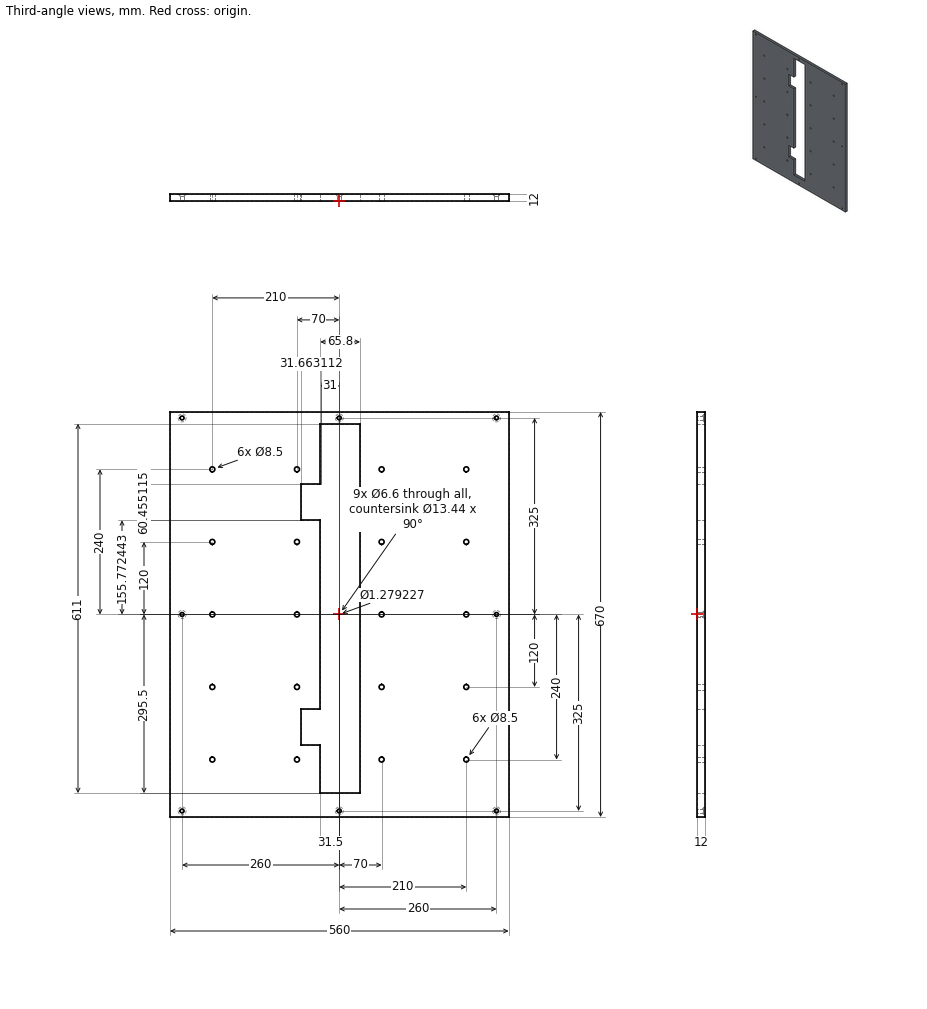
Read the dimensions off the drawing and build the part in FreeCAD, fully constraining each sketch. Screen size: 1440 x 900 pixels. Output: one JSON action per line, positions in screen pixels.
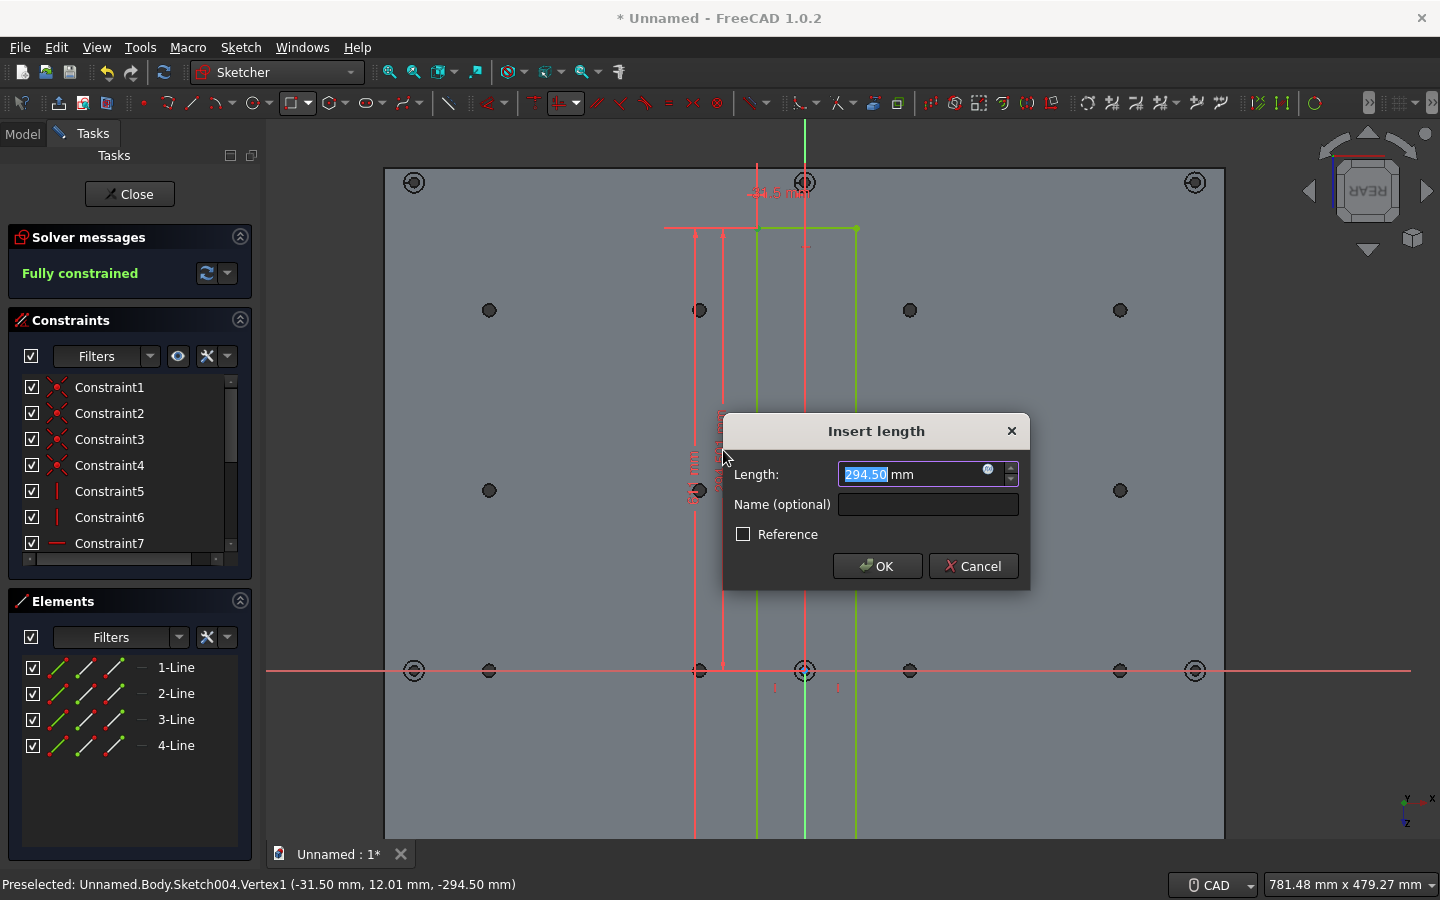
{"action": "type", "text": "295.5"}
{"action": "key", "text": "Return"}
{"action": "key", "text": "Escape"}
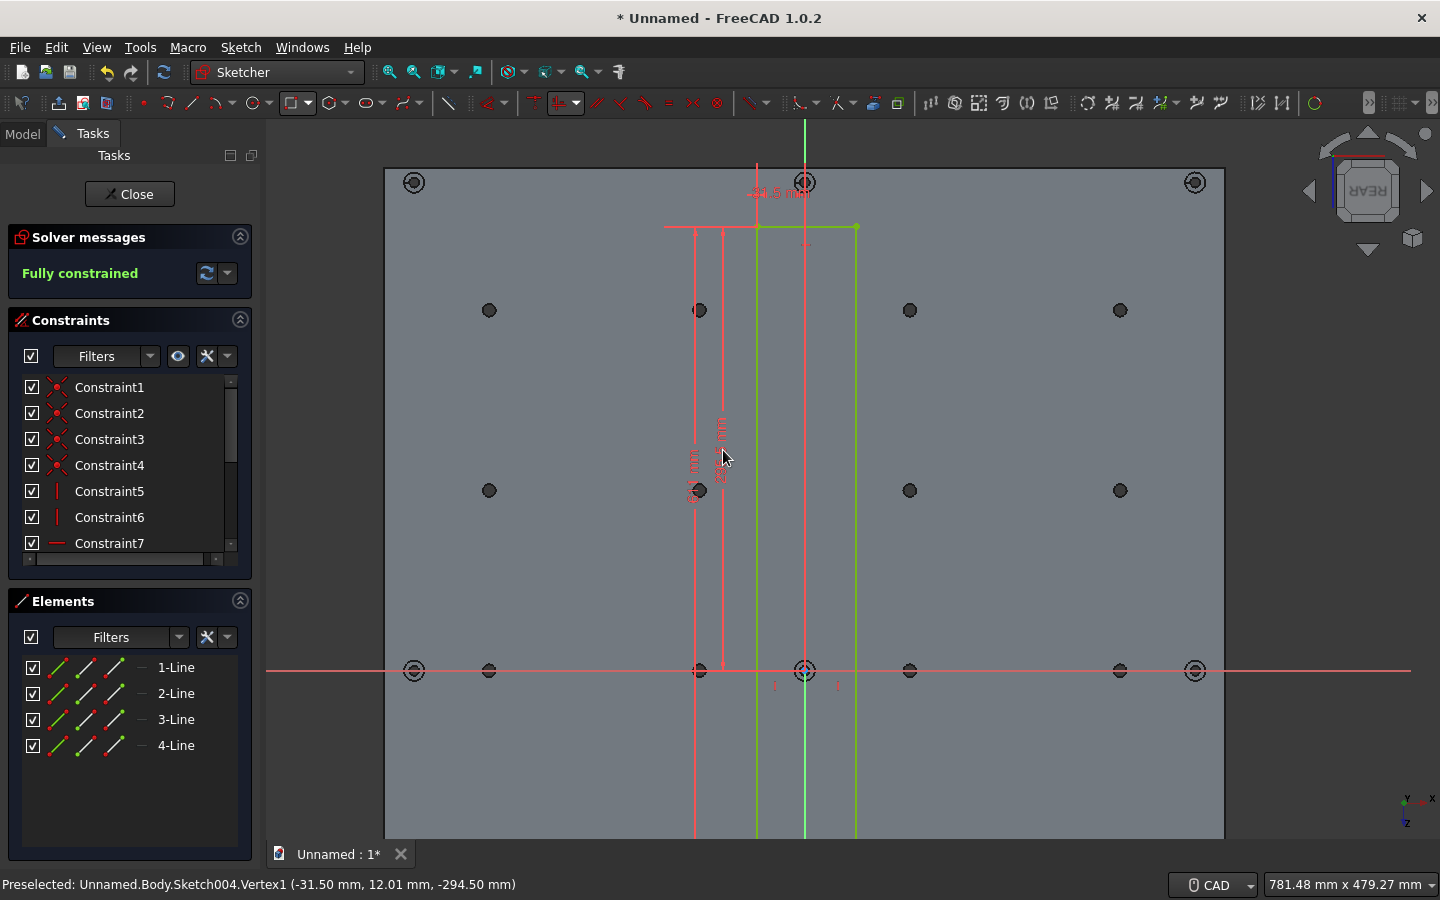
{"action": "left_click", "coordinate": [130, 194]}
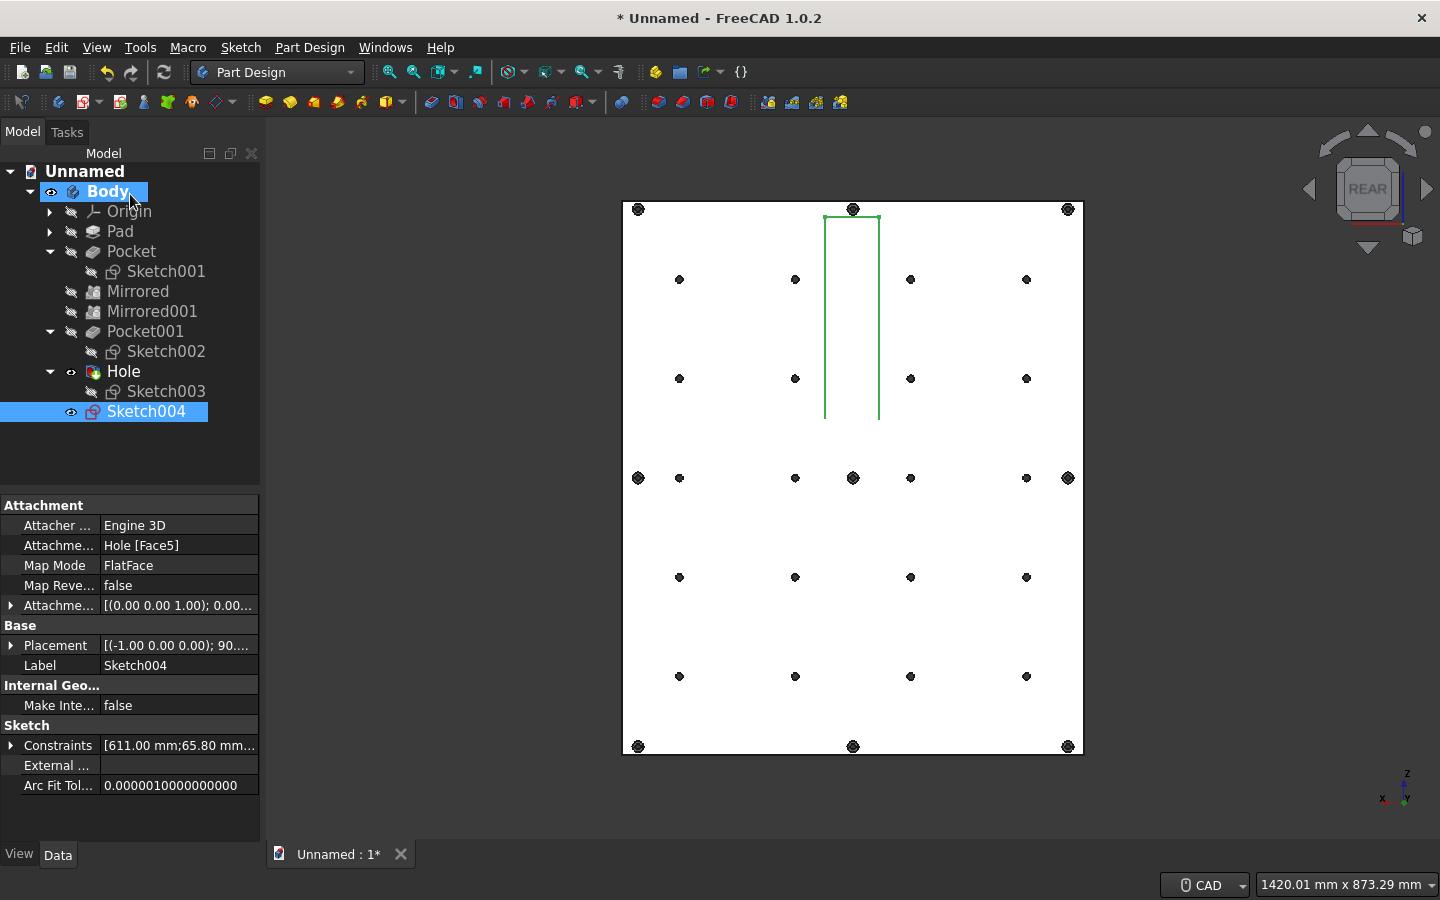
{"action": "left_click", "coordinate": [432, 102]}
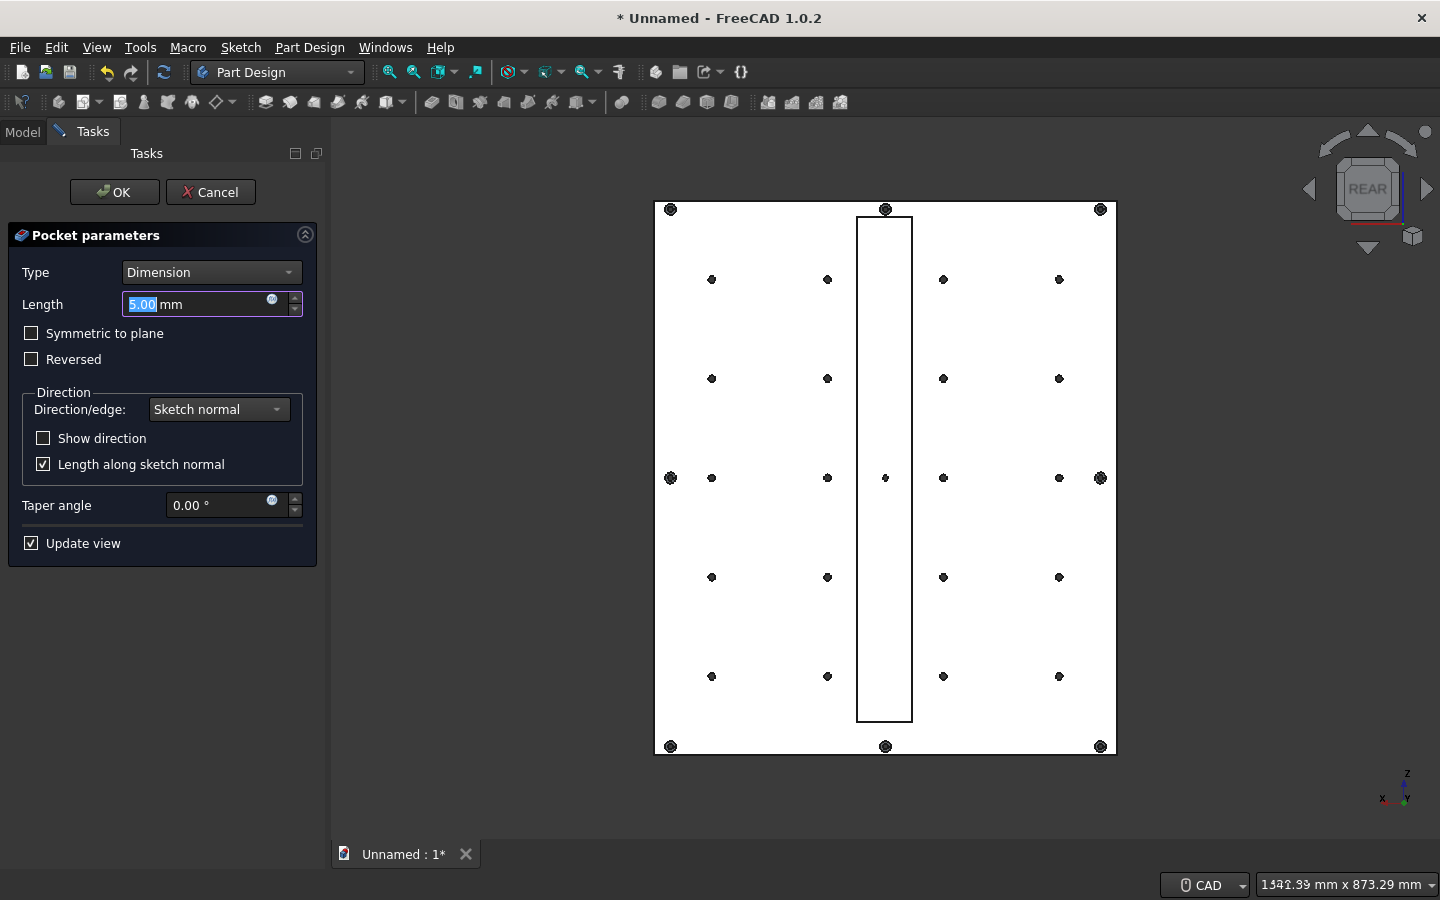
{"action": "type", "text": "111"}
{"action": "key", "text": "Tab"}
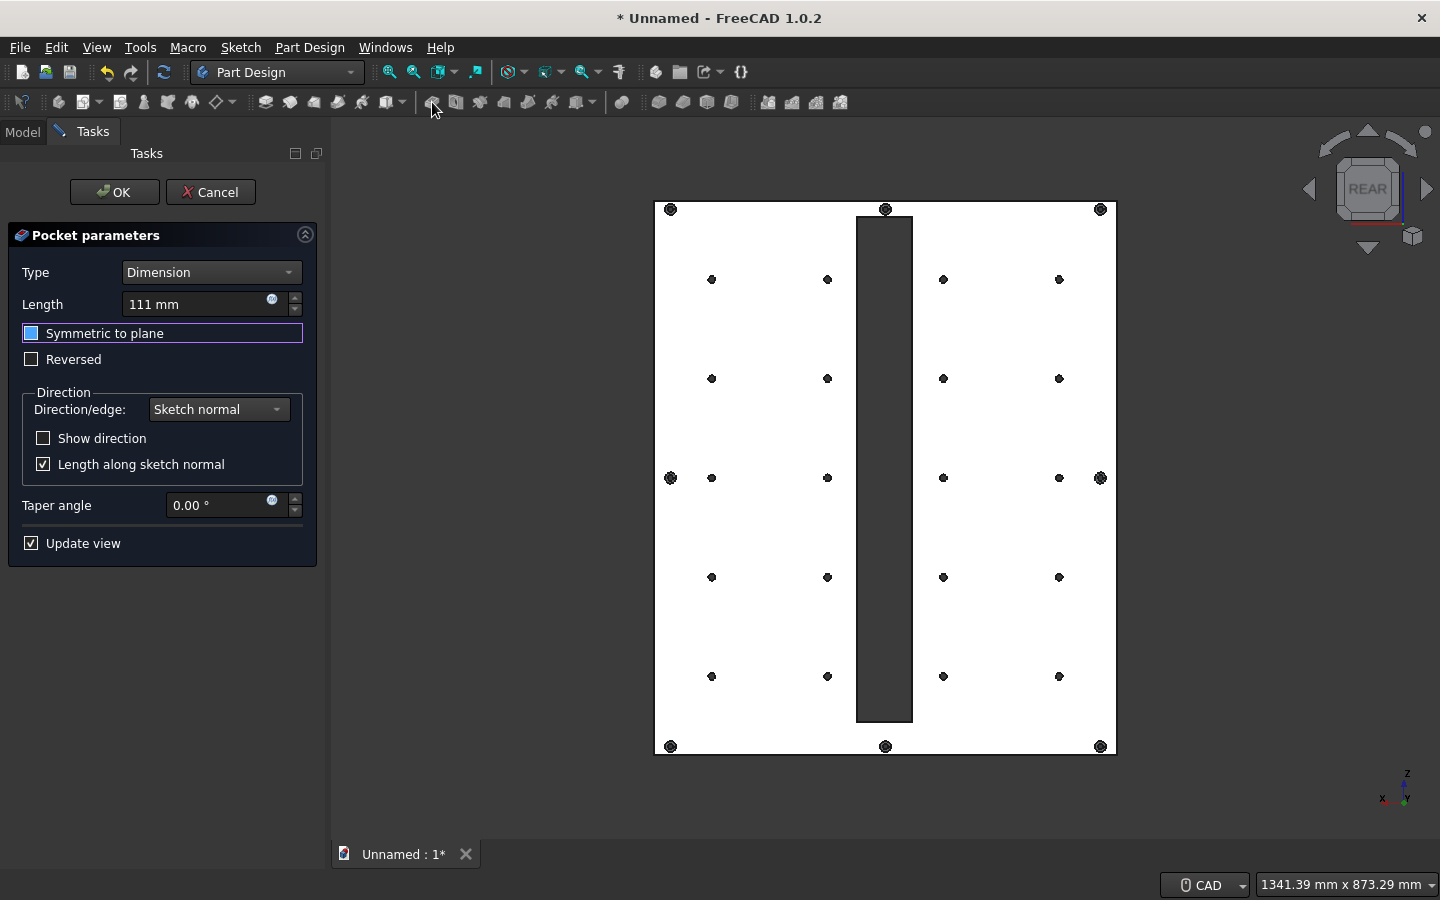
{"action": "left_click", "coordinate": [115, 192]}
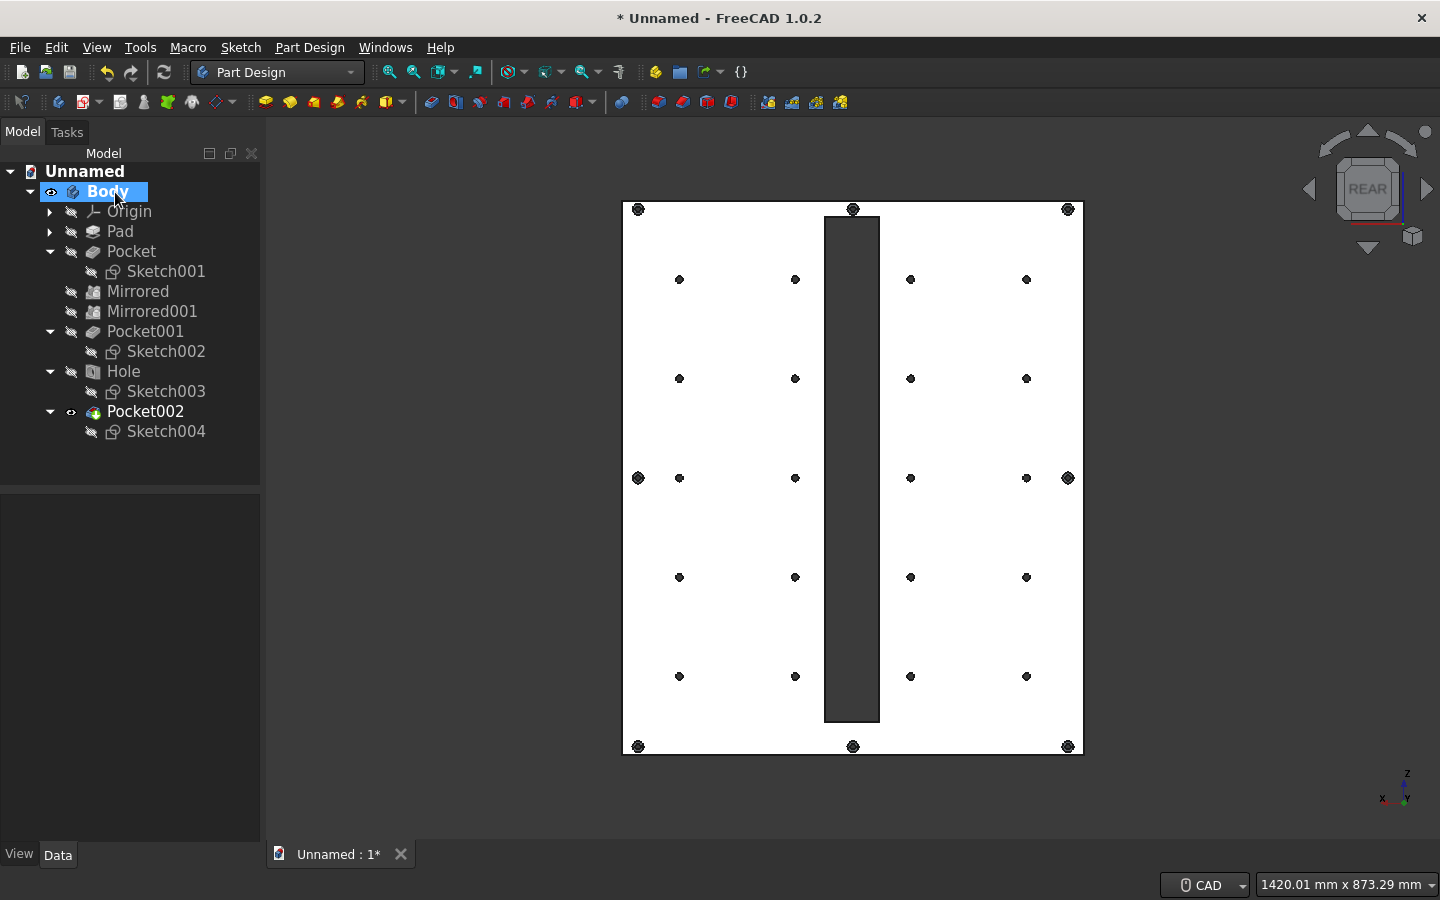
{"action": "left_click", "coordinate": [721, 635]}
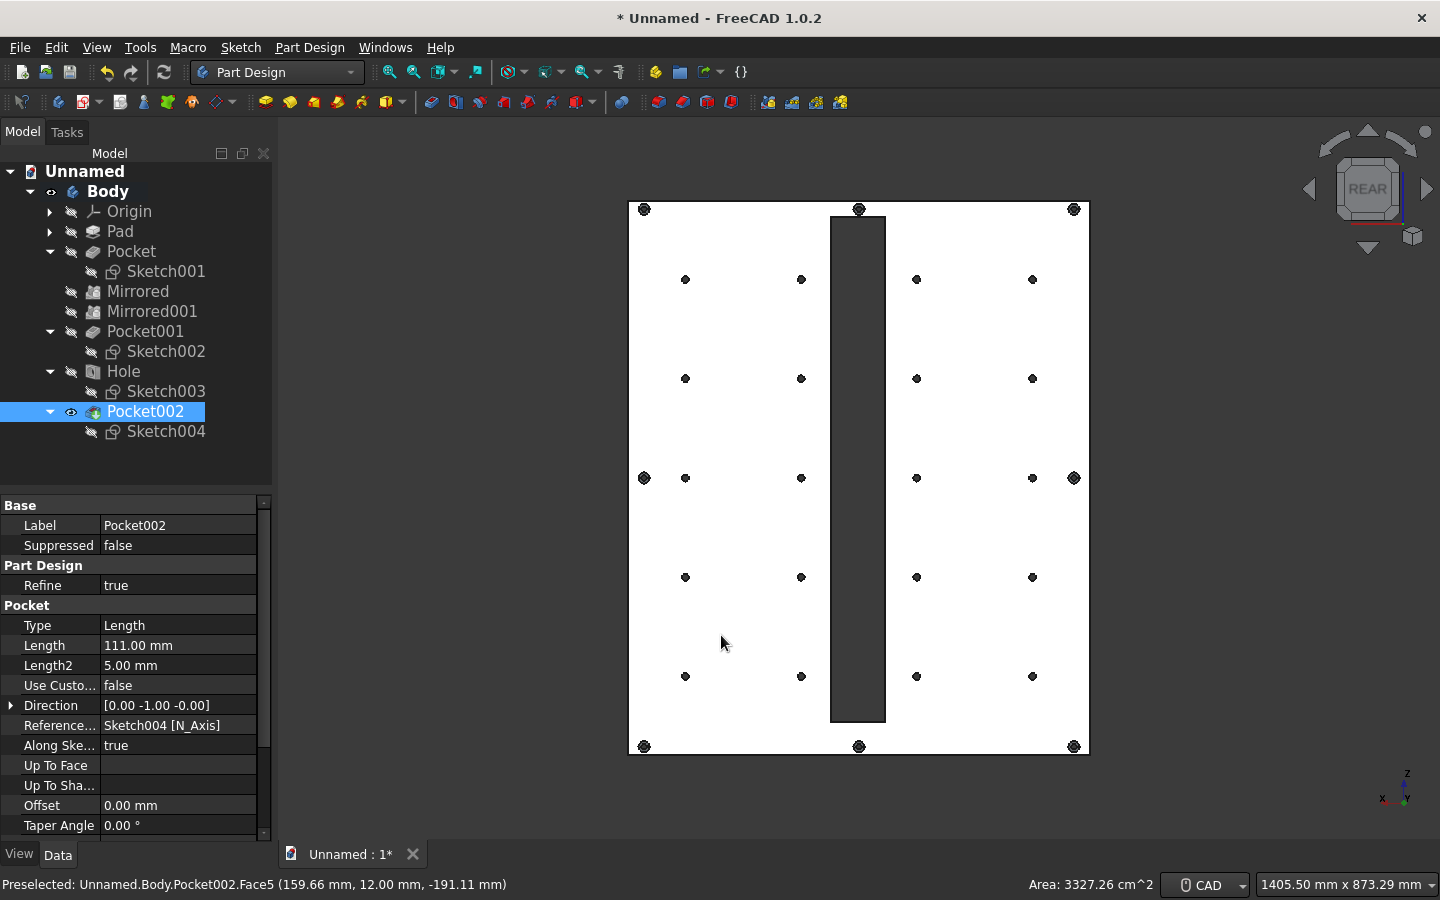
{"action": "left_click", "coordinate": [84, 102]}